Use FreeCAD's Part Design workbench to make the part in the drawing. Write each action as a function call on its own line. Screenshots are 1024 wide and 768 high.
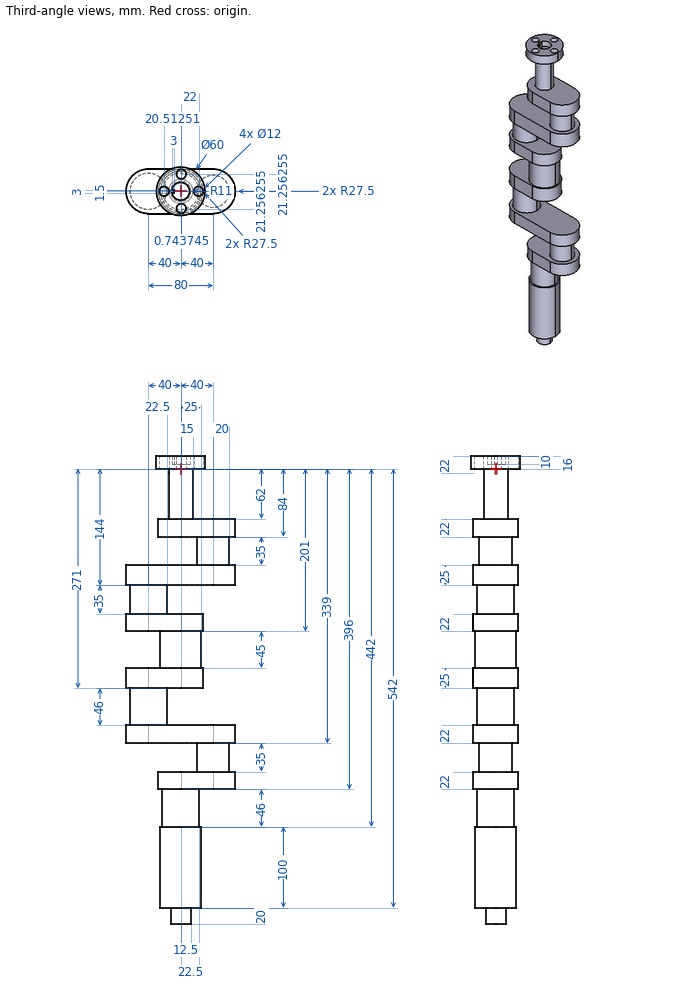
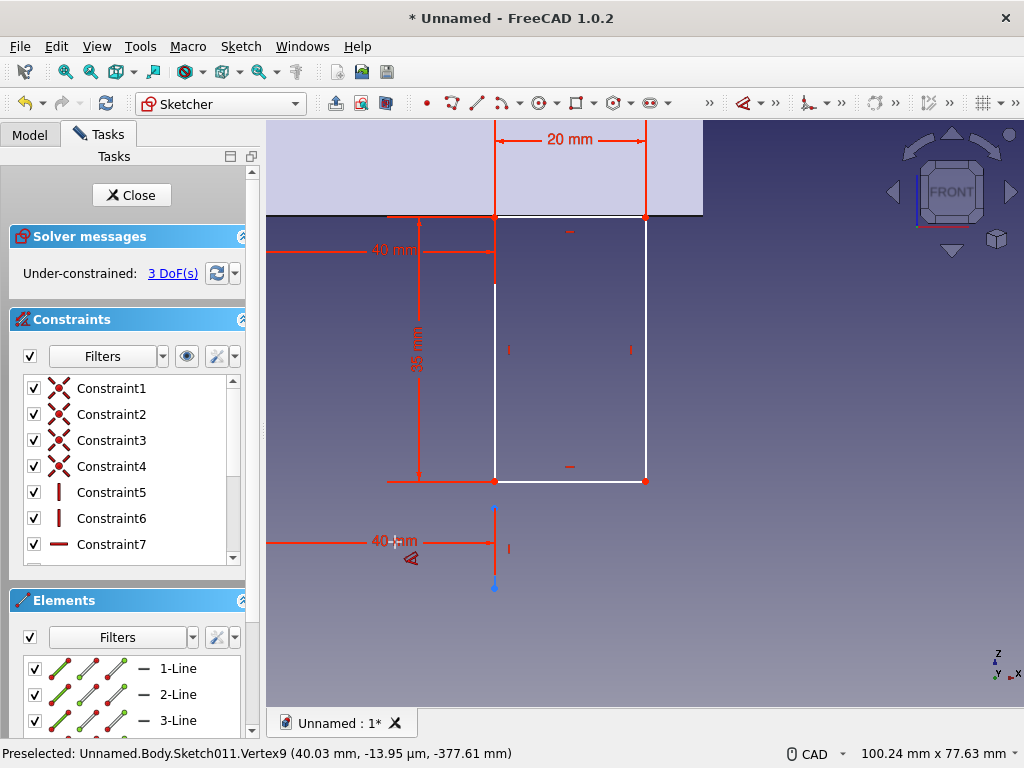
click(495, 217)
click(529, 183)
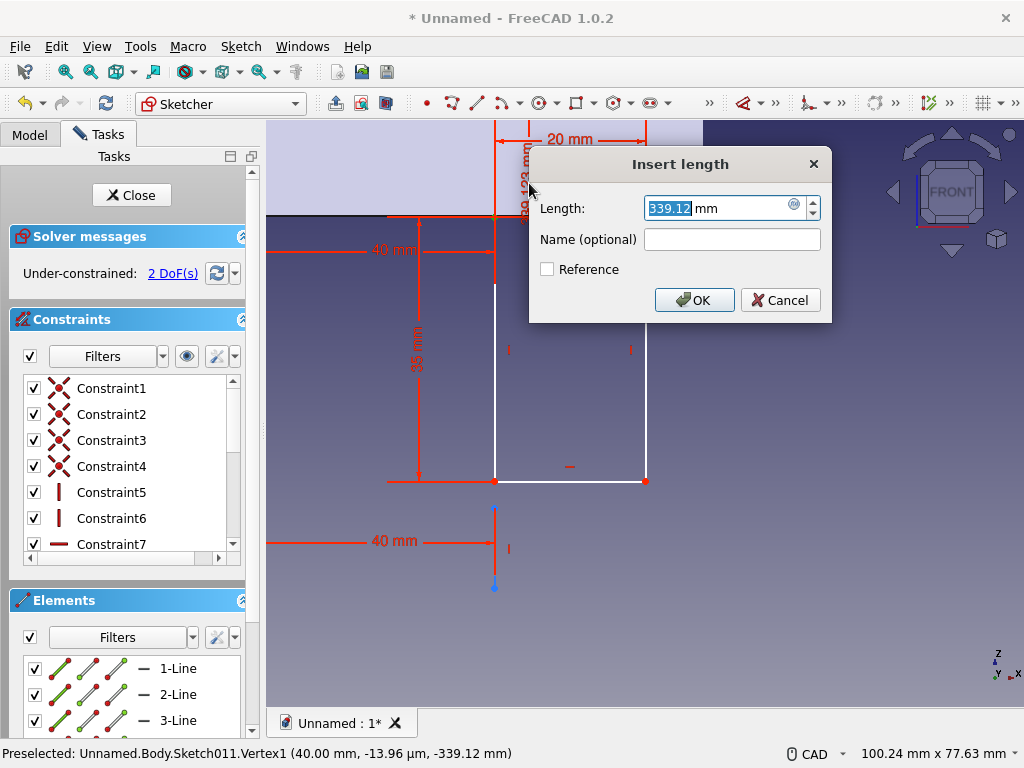
text(339)
key(Return)
key(Escape)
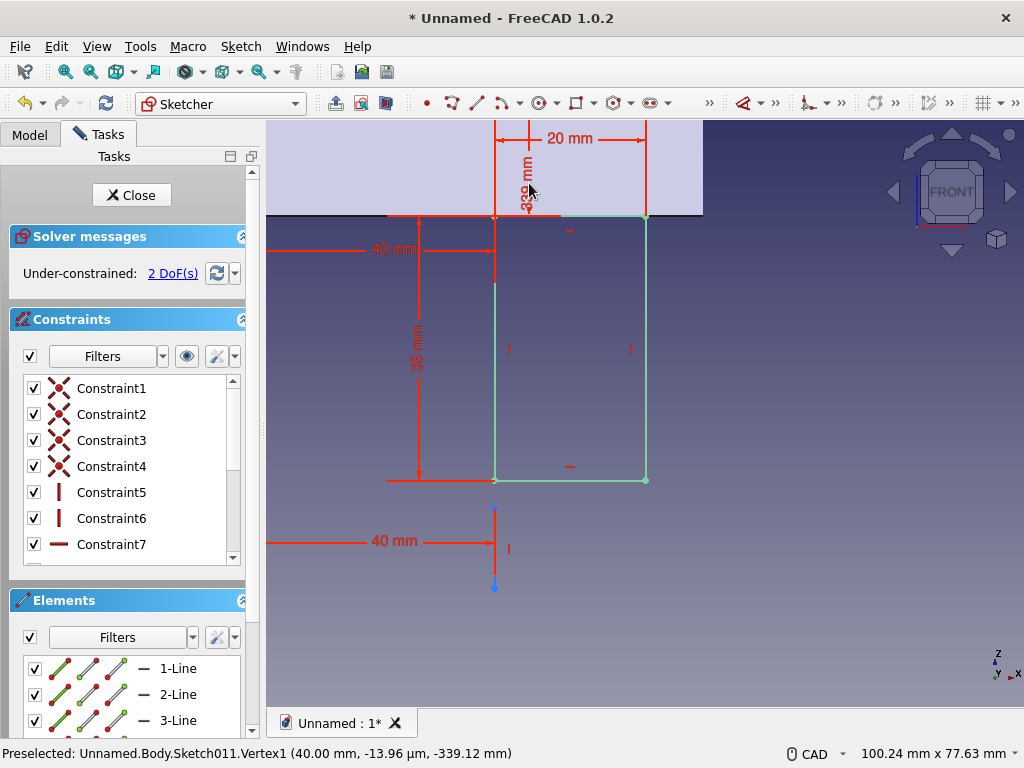
click(132, 195)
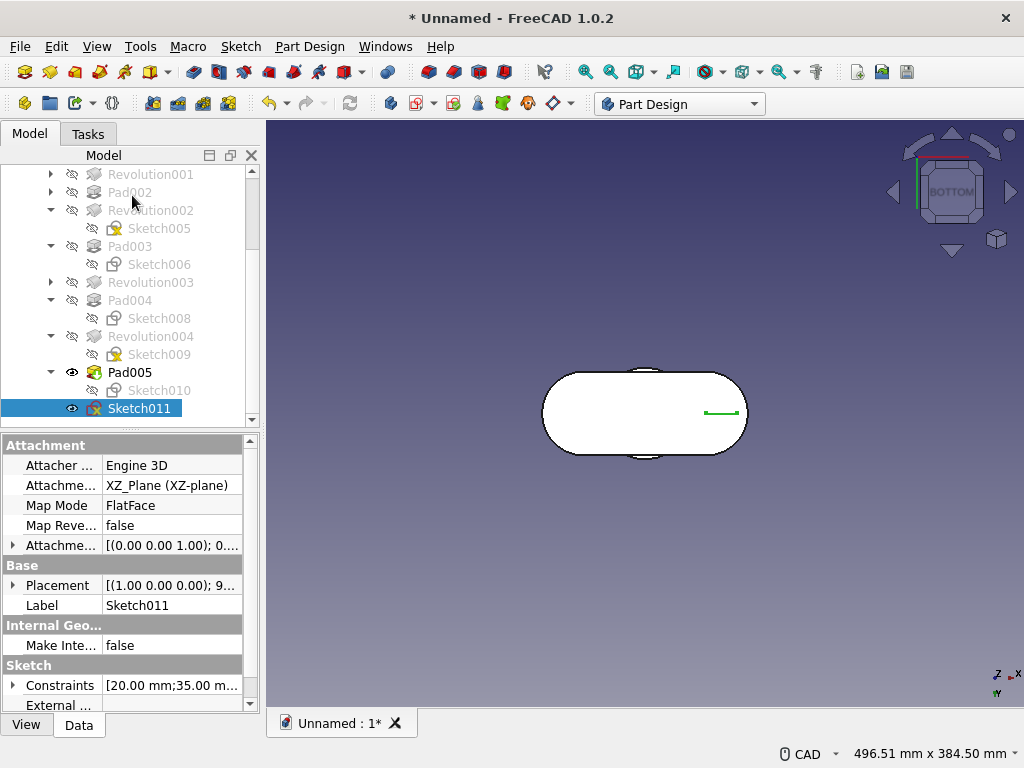
click(50, 72)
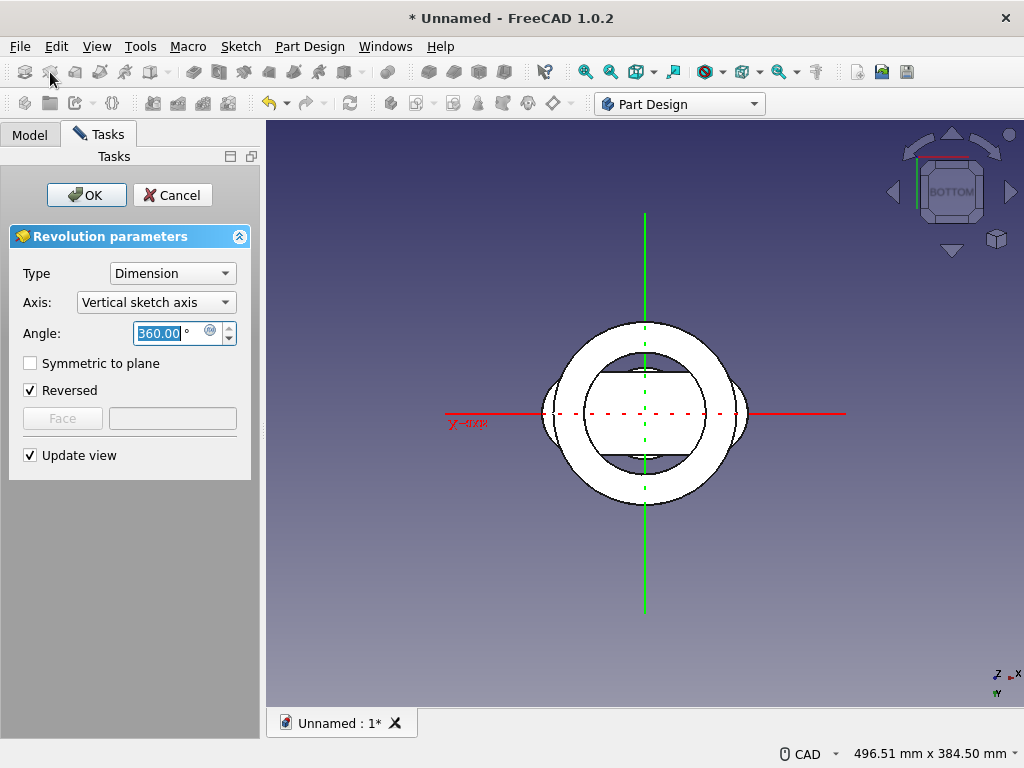
click(157, 302)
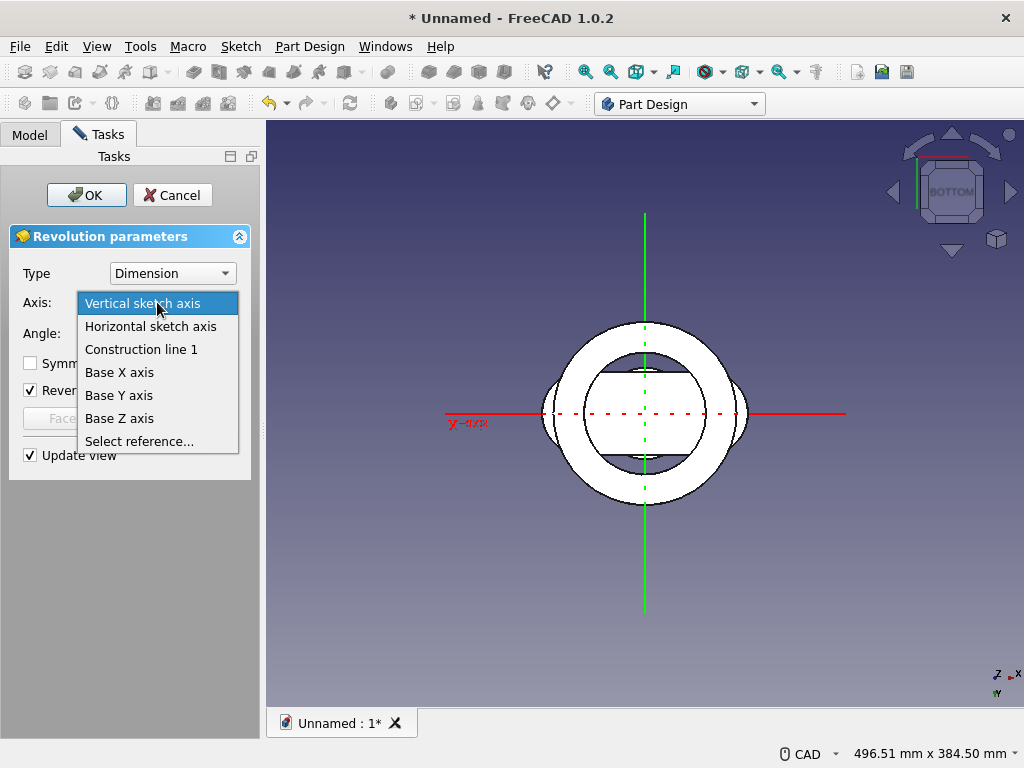
click(156, 350)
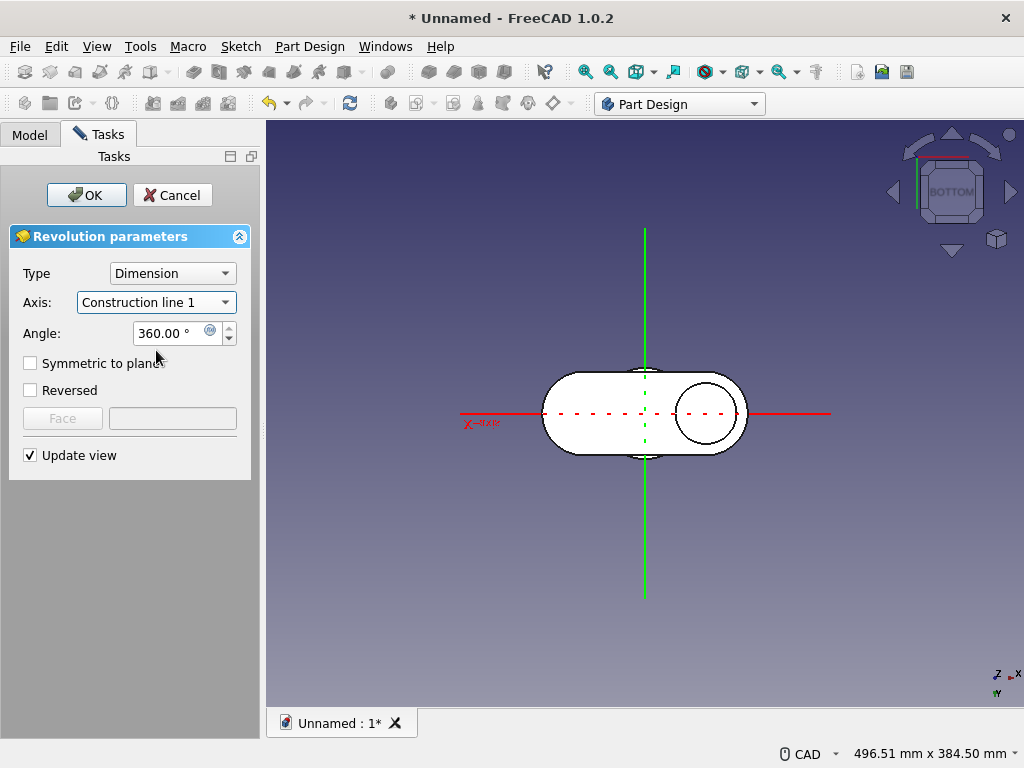
click(87, 195)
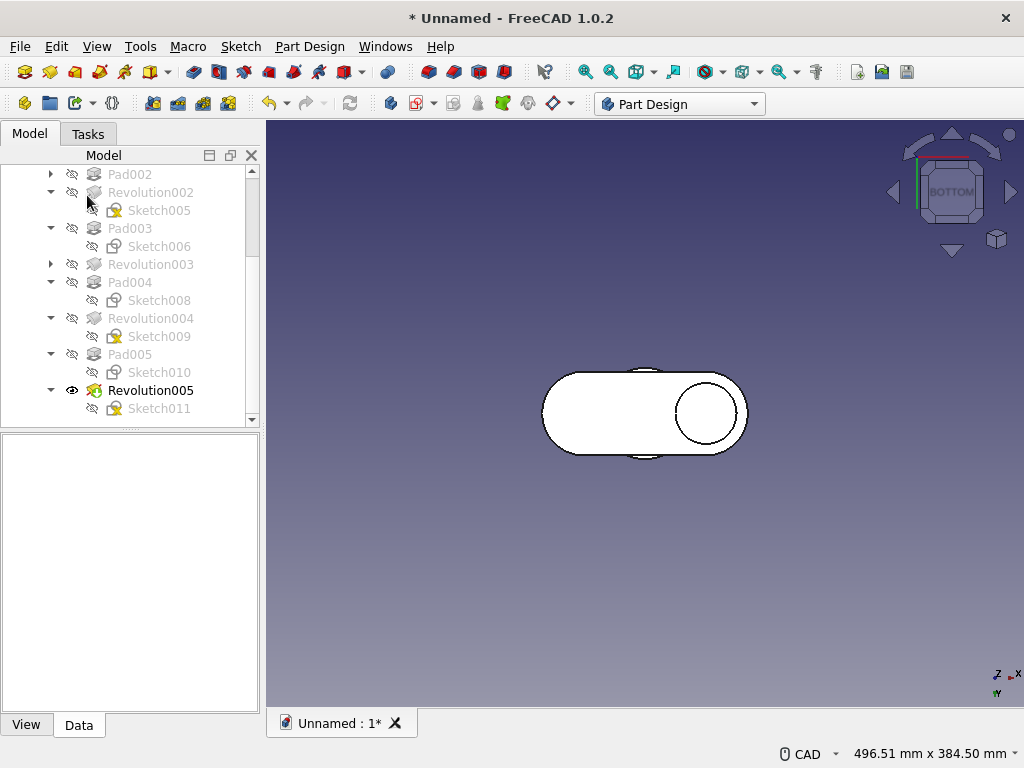
key(v)
key(f)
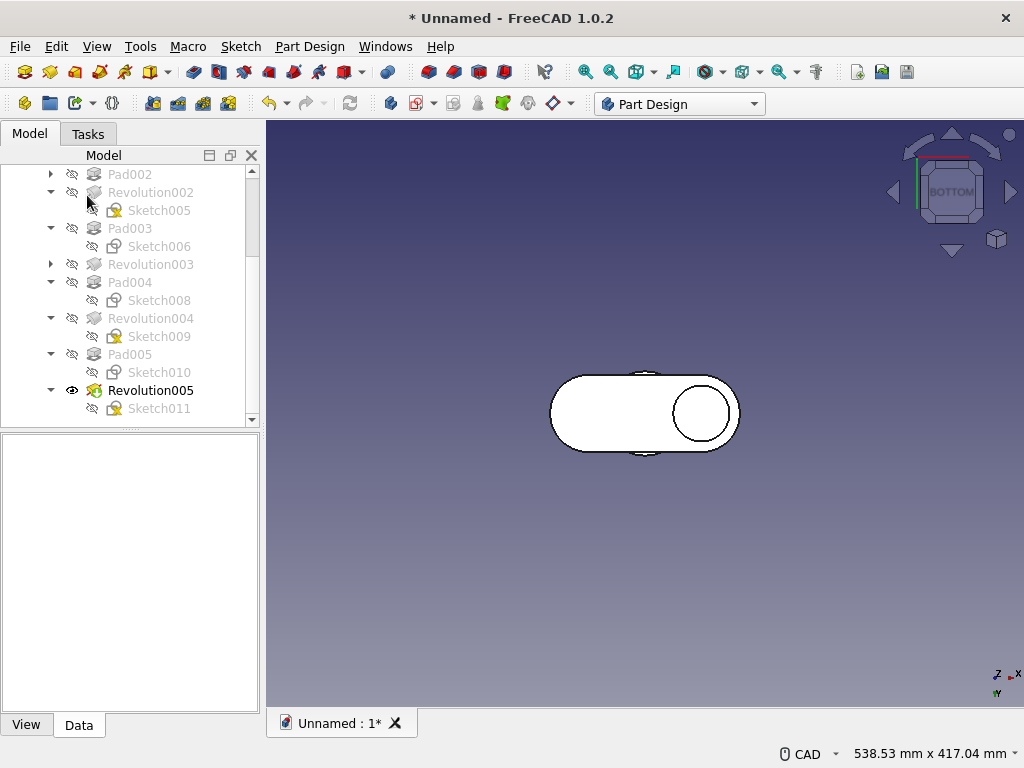
click(701, 412)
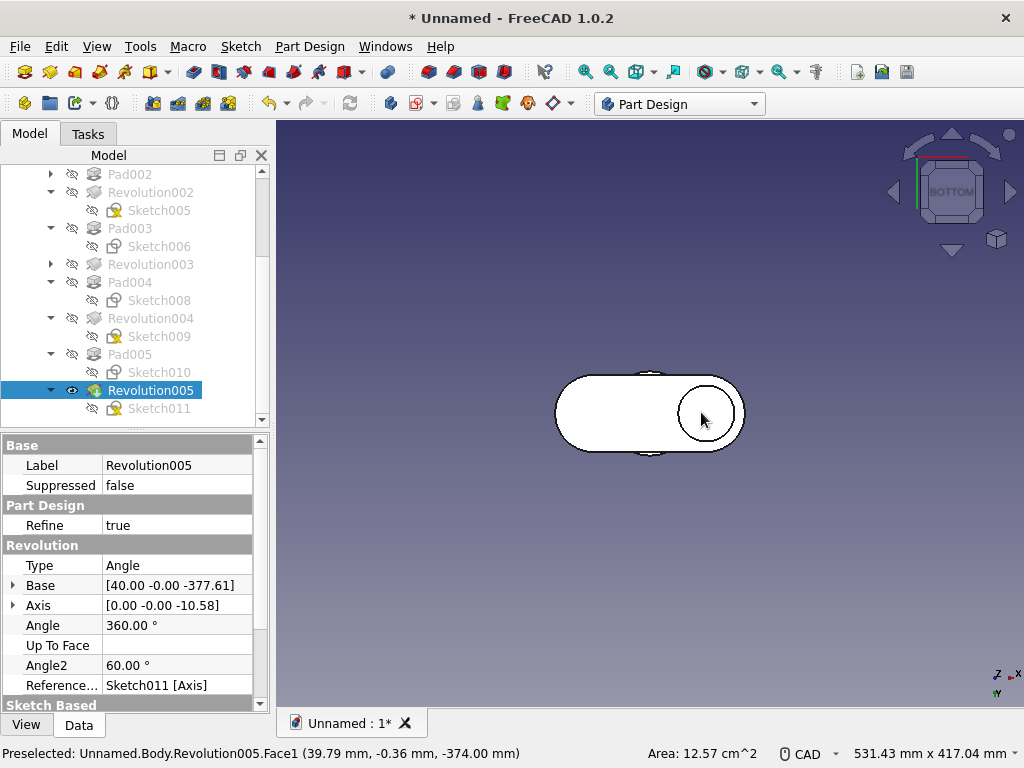
click(416, 104)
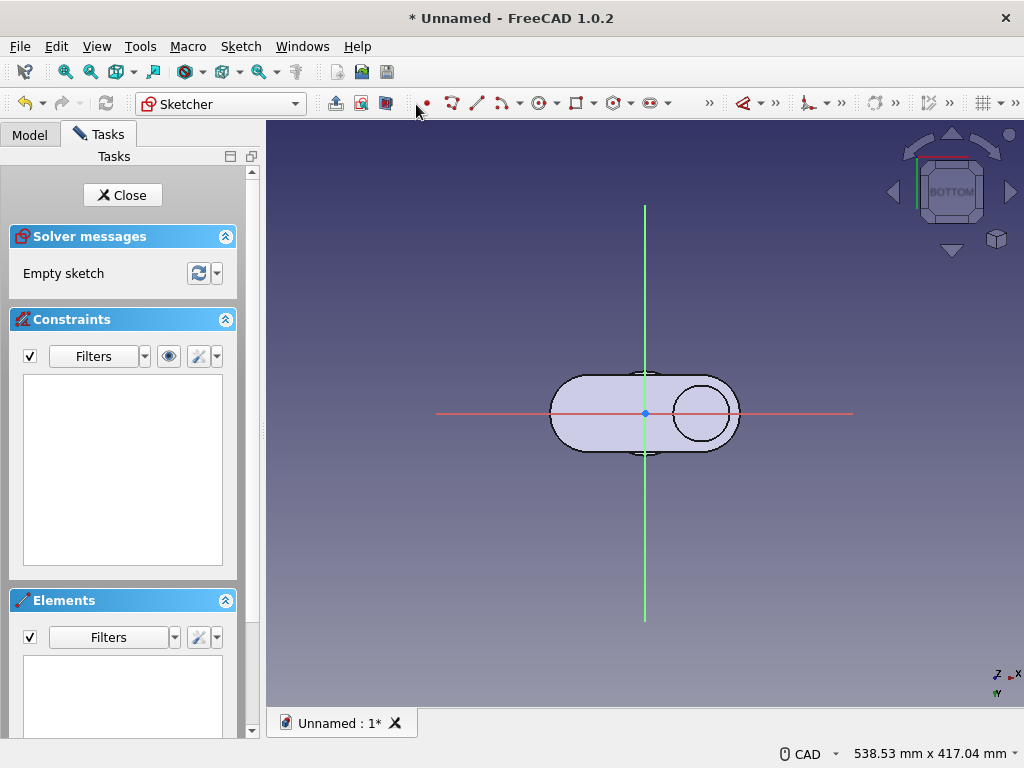
scroll(729, 413, up, 5)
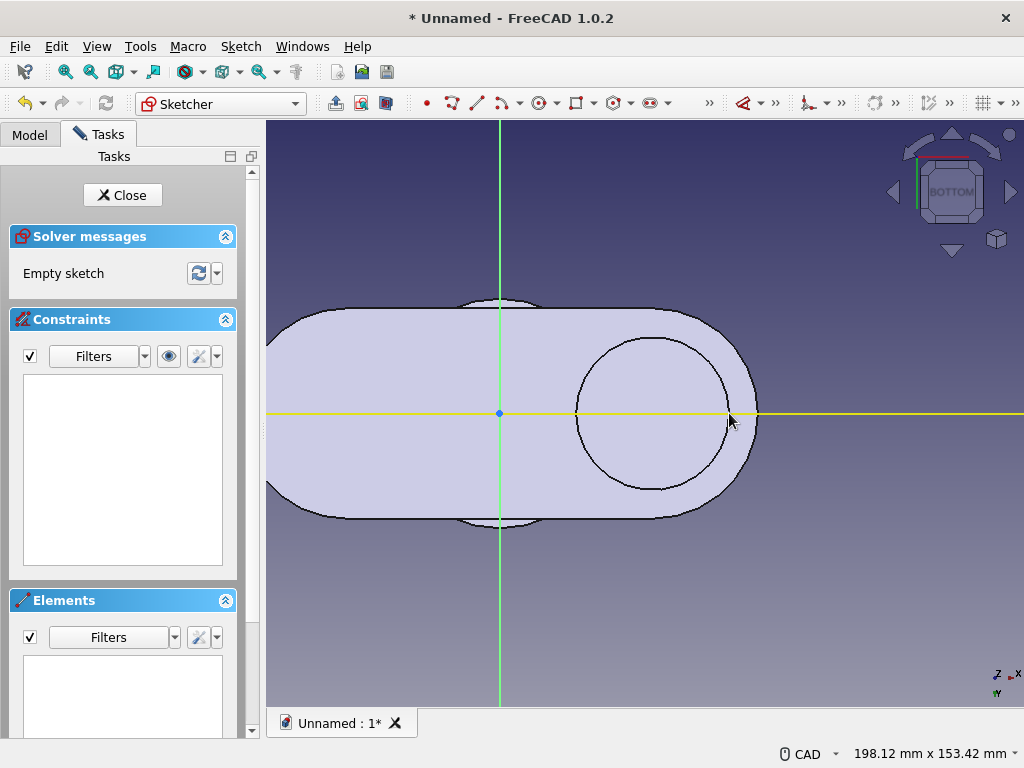
key(g)
key(s)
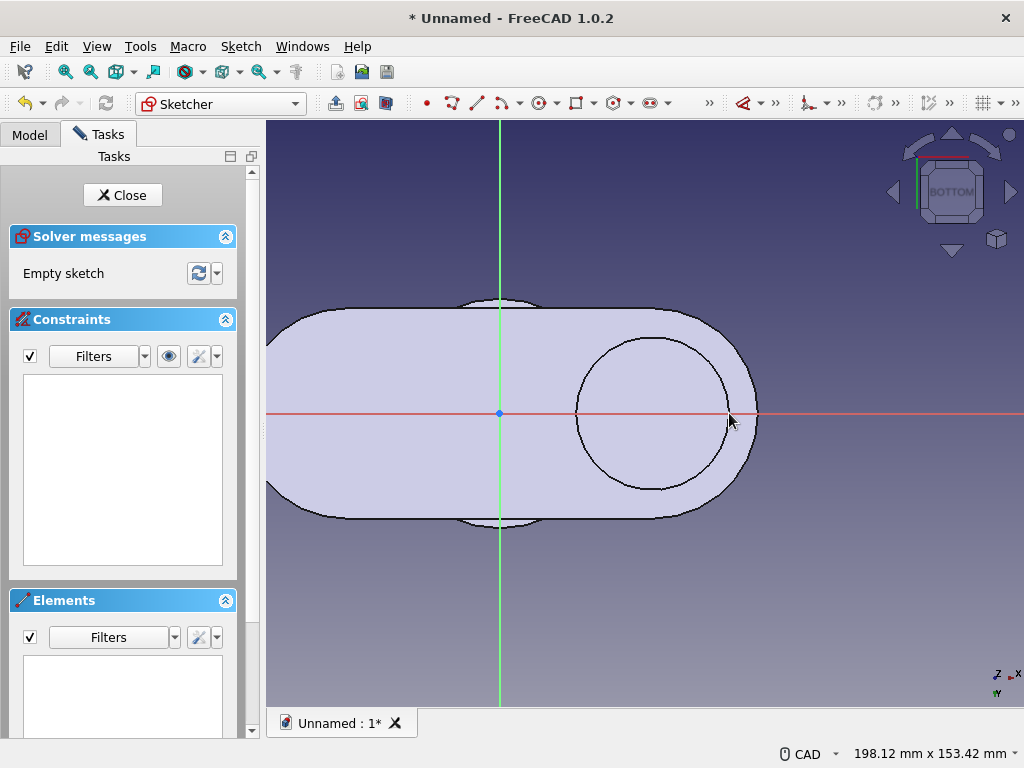
click(500, 413)